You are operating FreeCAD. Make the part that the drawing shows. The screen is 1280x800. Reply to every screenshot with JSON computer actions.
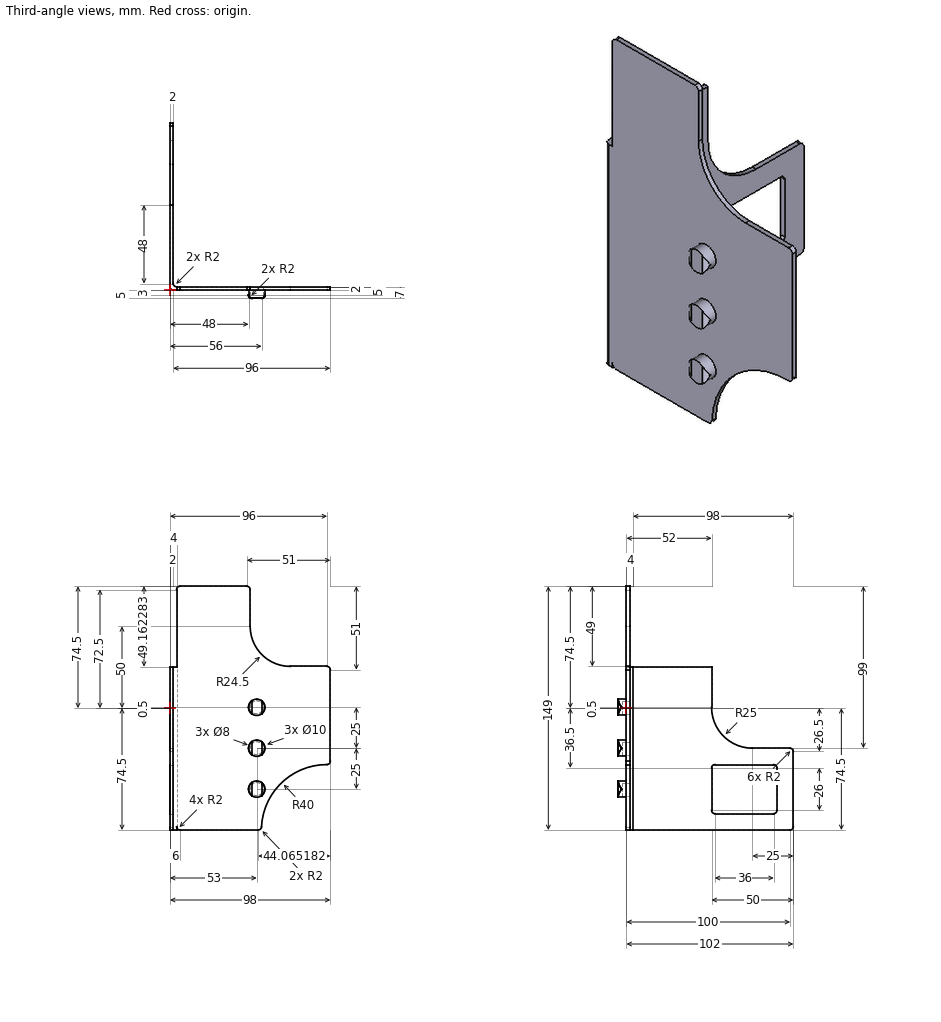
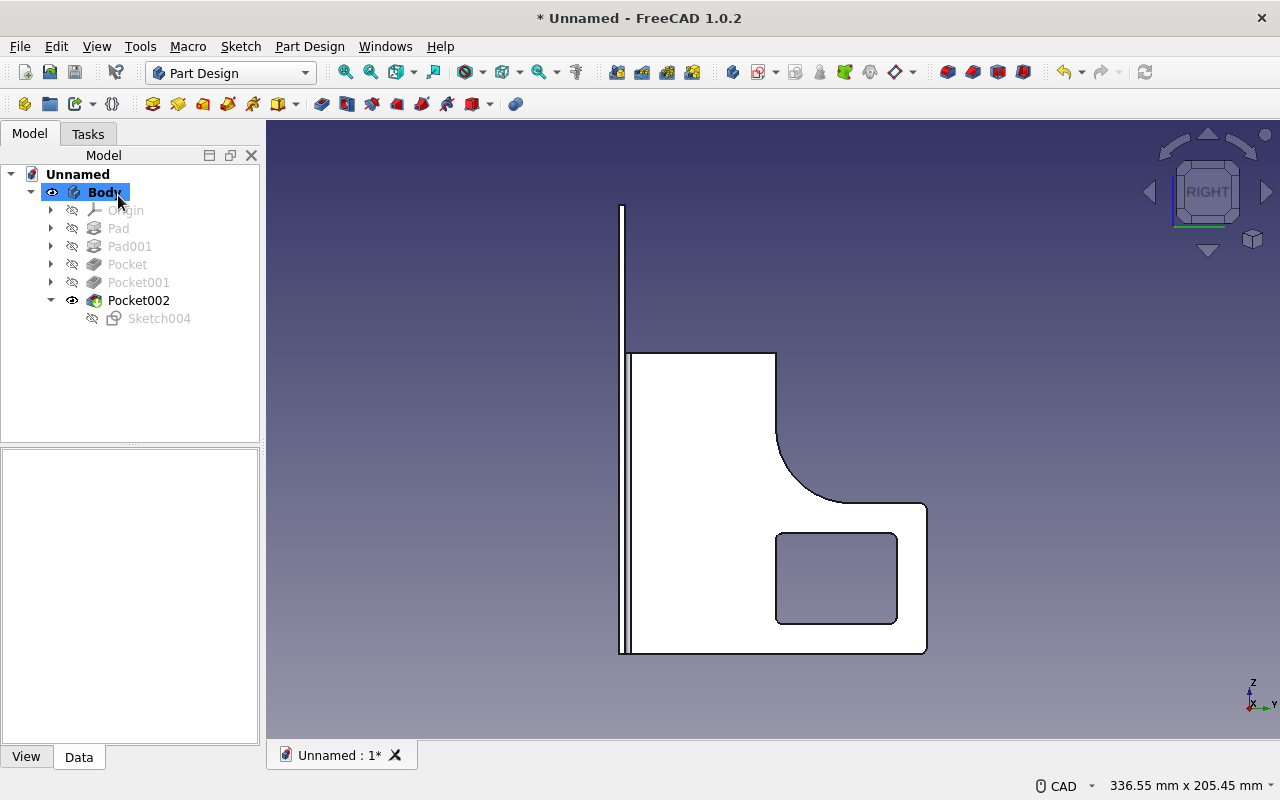
{"action": "key", "text": "4"}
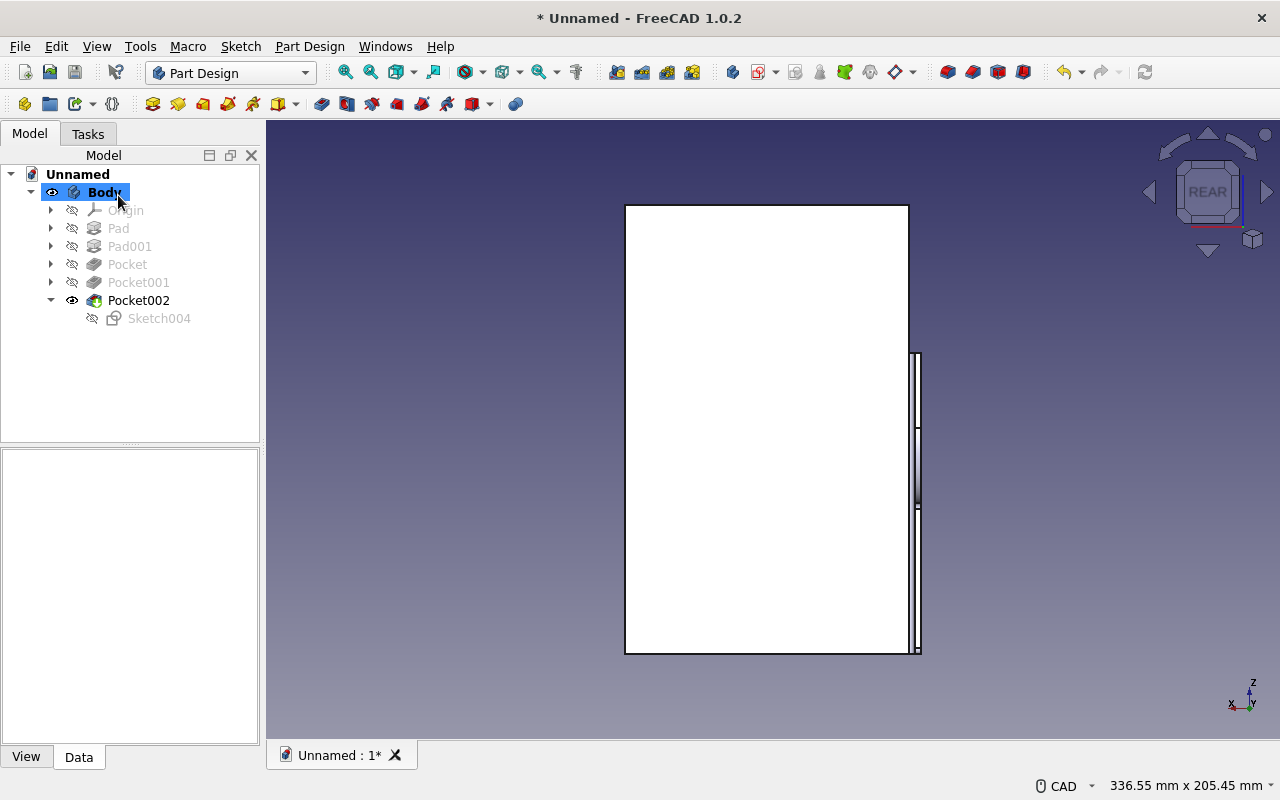
{"action": "left_click", "coordinate": [767, 364]}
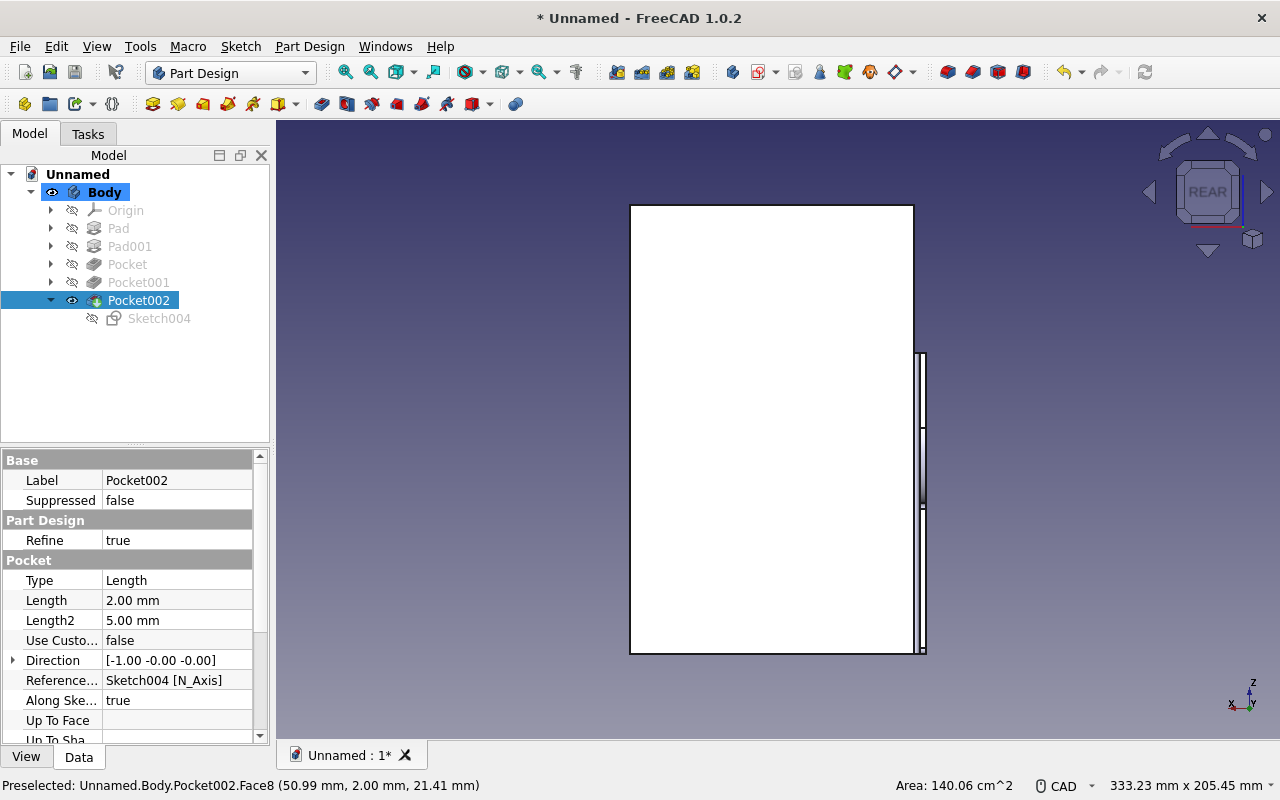
{"action": "left_click", "coordinate": [758, 72]}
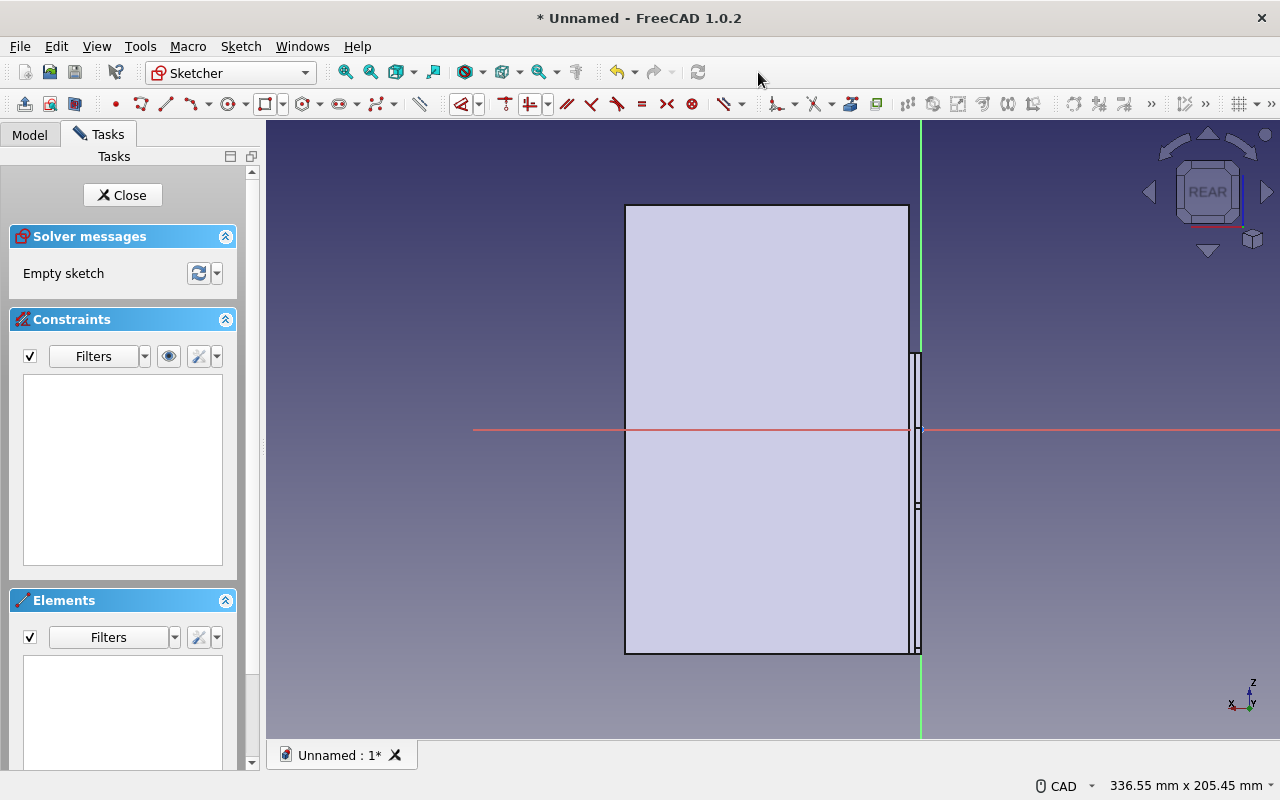
{"action": "left_click", "coordinate": [75, 104]}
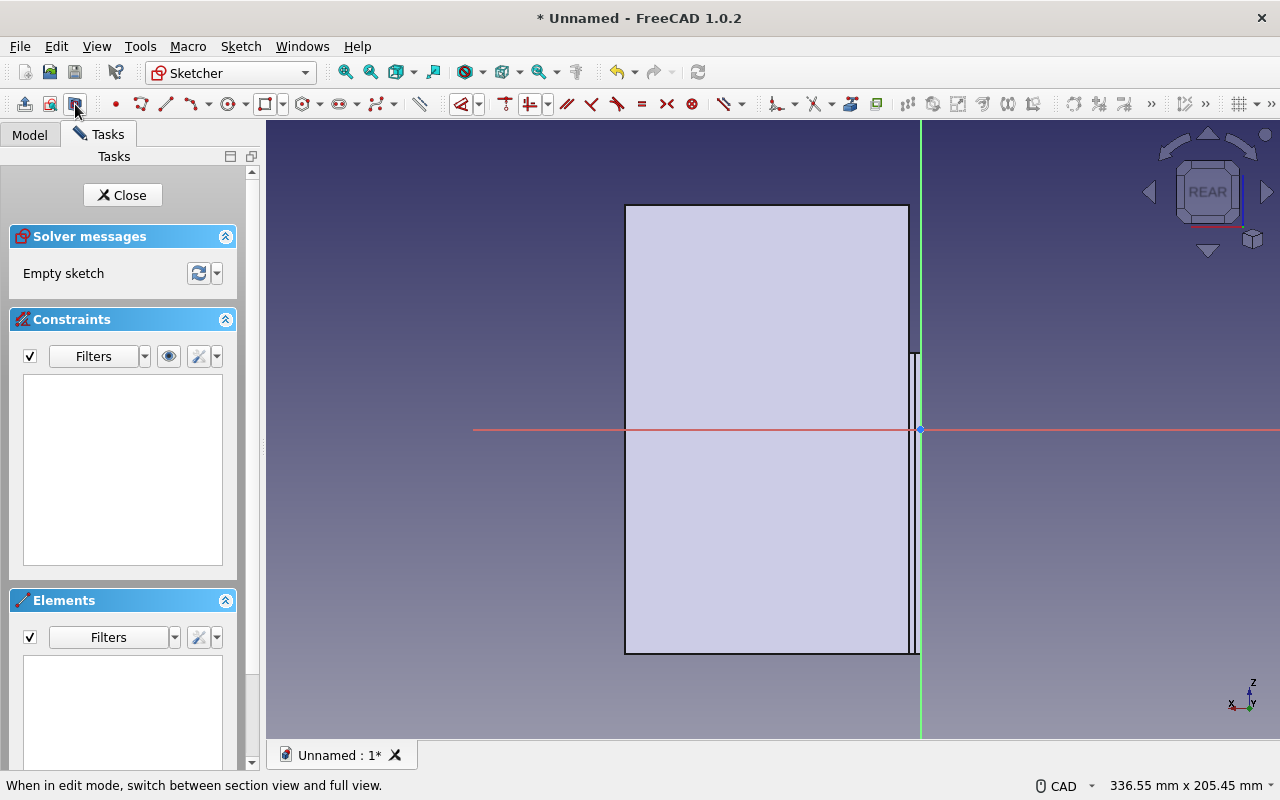
{"action": "left_click", "coordinate": [141, 104]}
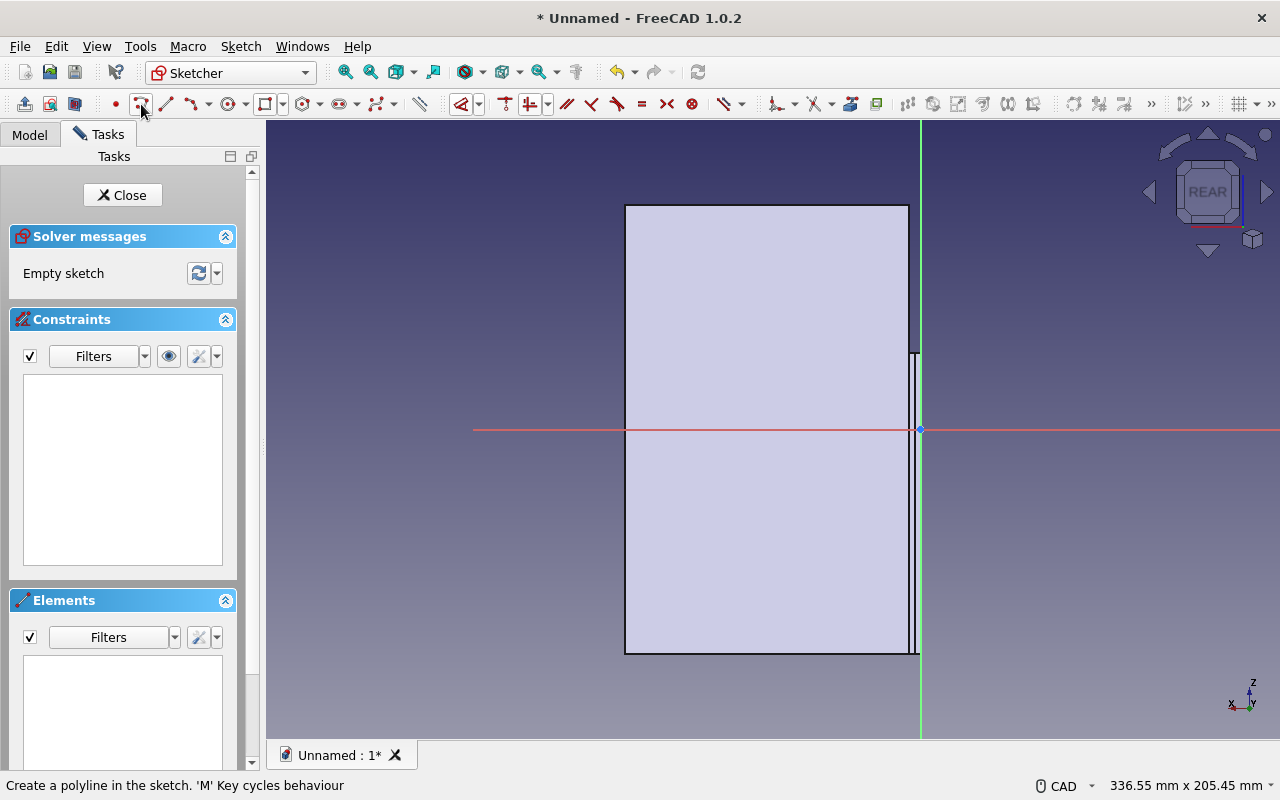
{"action": "left_click", "coordinate": [903, 654]}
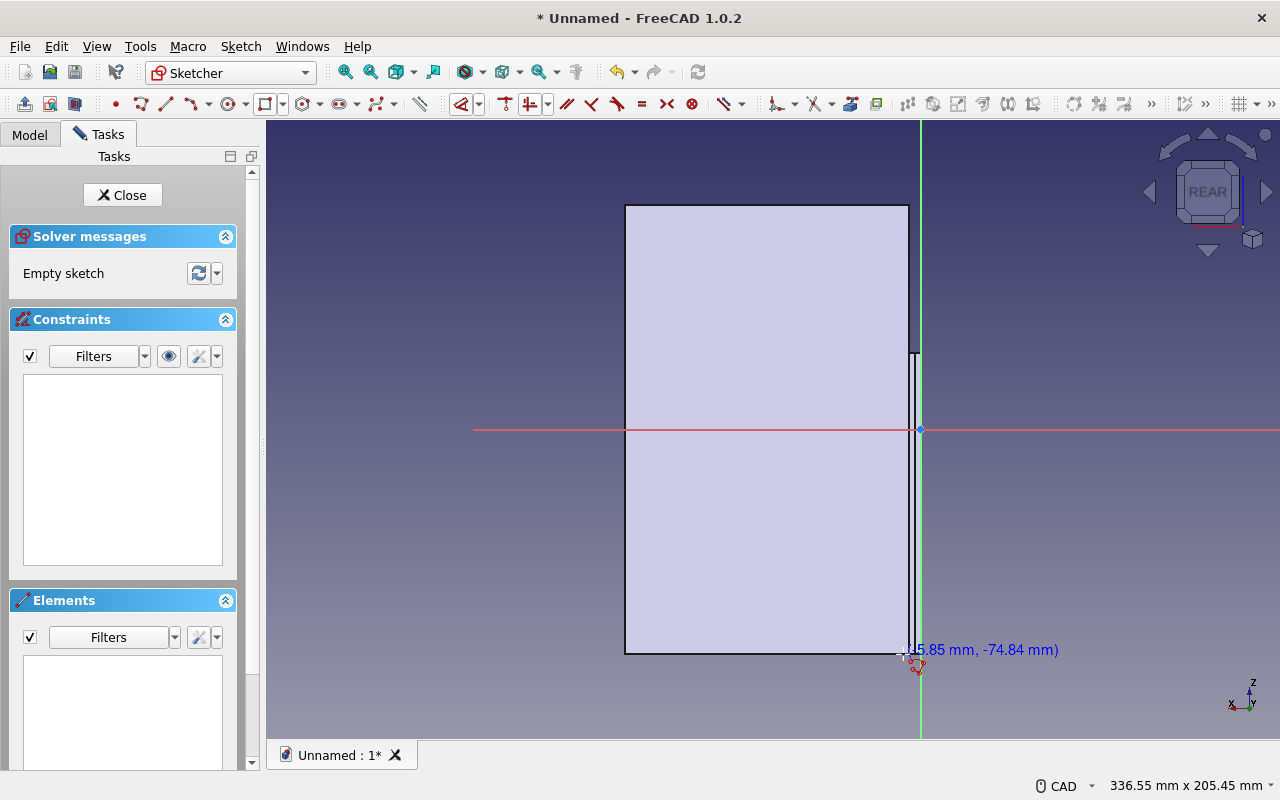
{"action": "scroll", "coordinate": [909, 654], "scroll_direction": "up", "scroll_amount": 5}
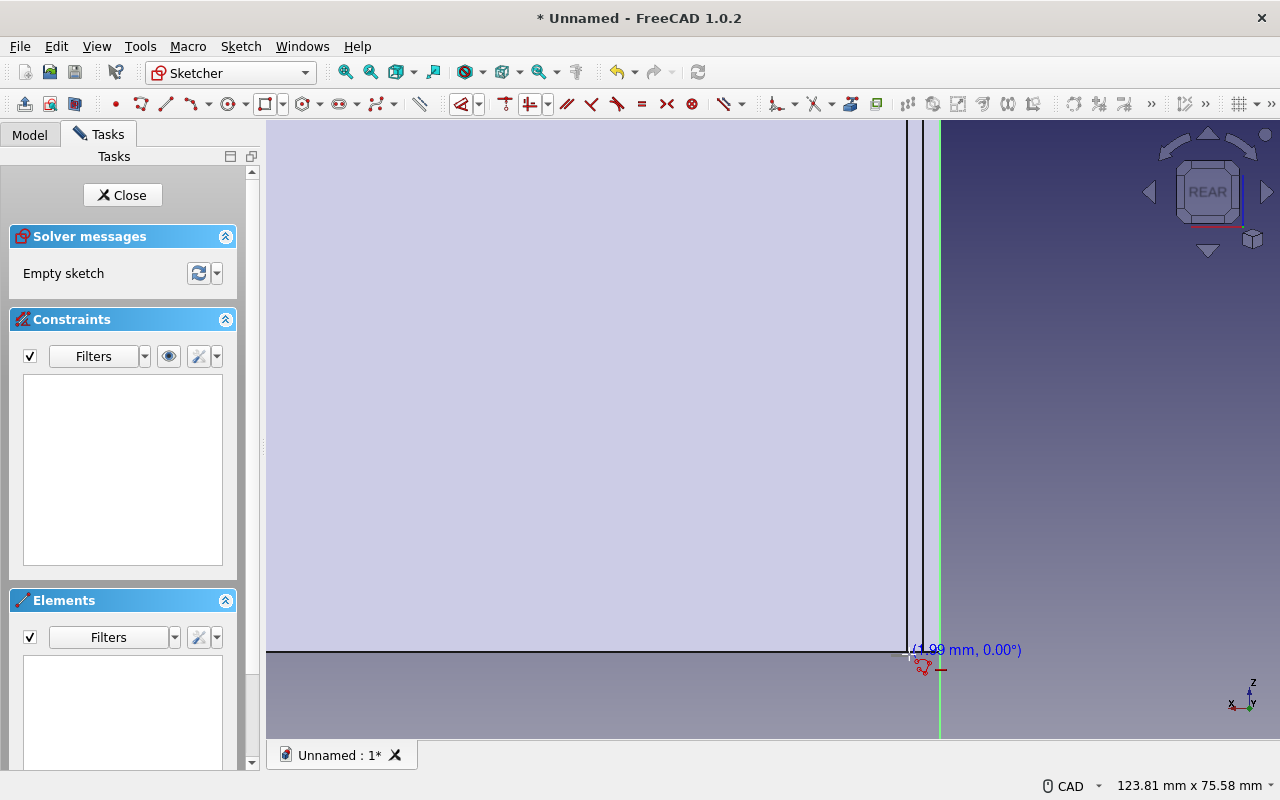
{"action": "left_click", "coordinate": [907, 653]}
{"action": "left_click", "coordinate": [907, 636]}
{"action": "right_click", "coordinate": [907, 636]}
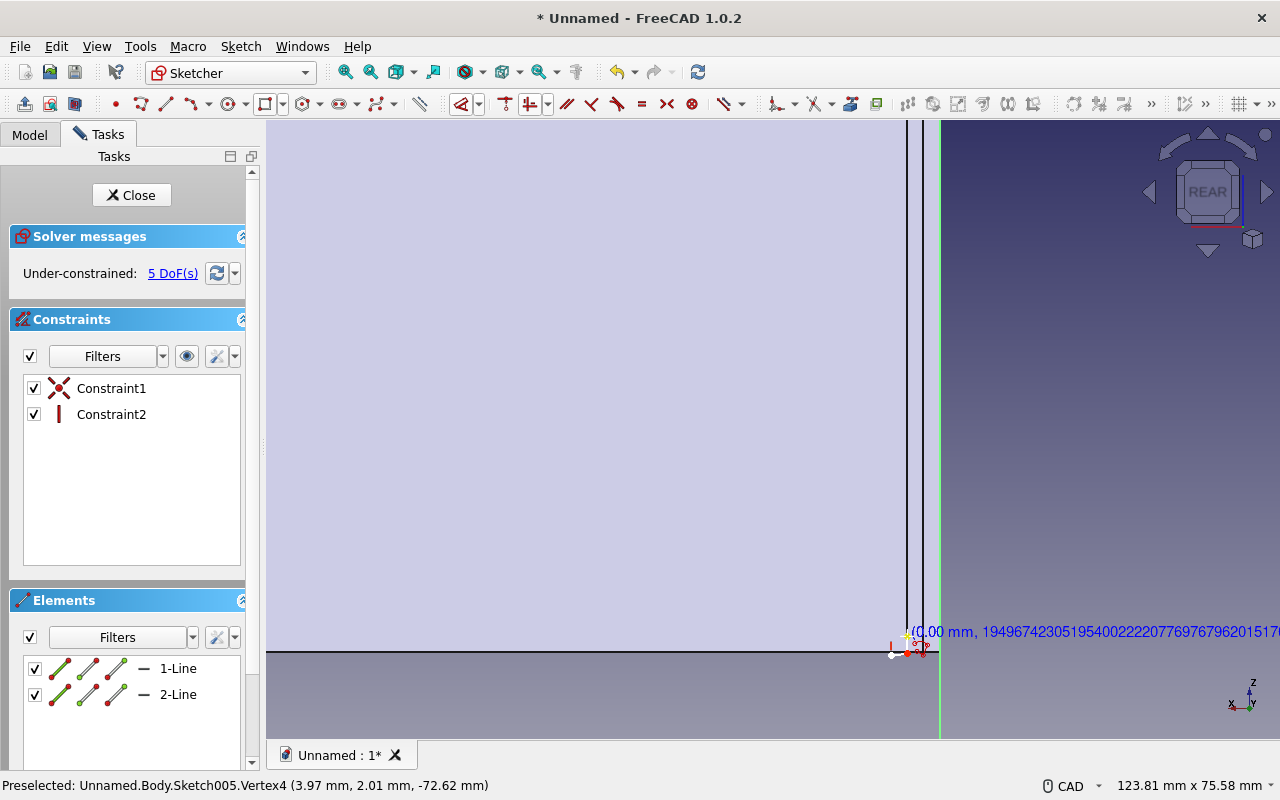
{"action": "key", "text": "g 3 a"}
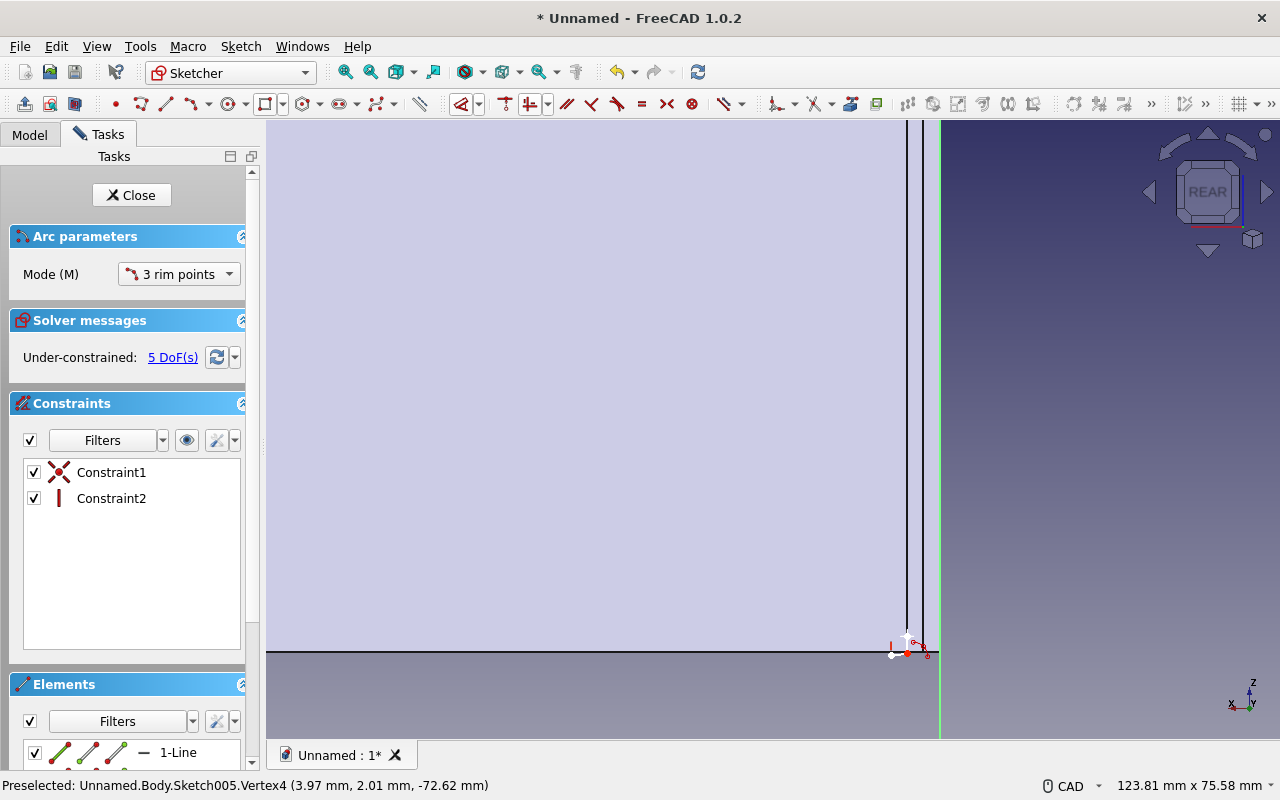
{"action": "scroll", "coordinate": [907, 636], "scroll_direction": "up", "scroll_amount": 4}